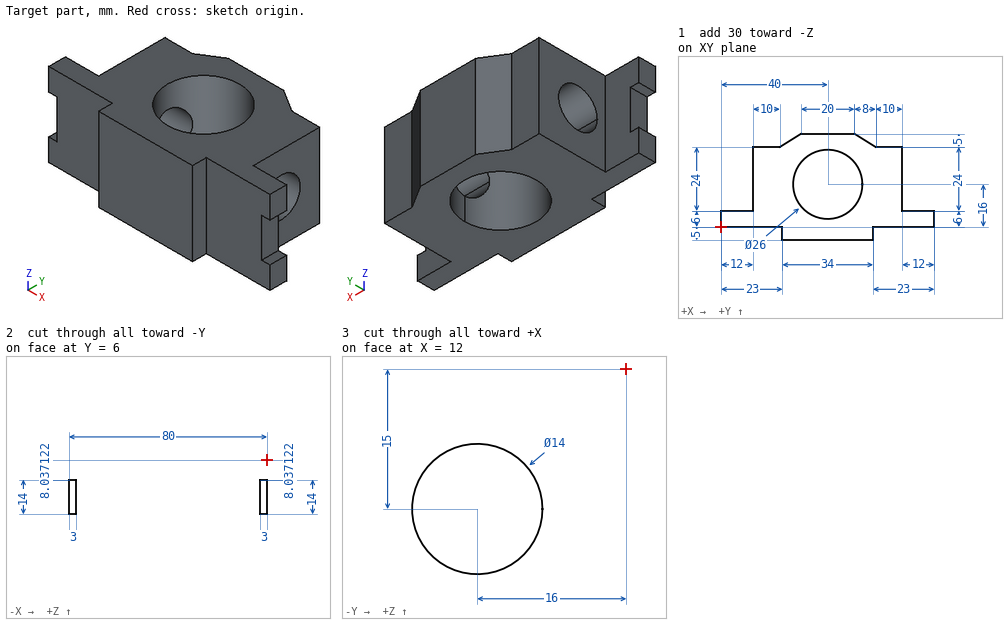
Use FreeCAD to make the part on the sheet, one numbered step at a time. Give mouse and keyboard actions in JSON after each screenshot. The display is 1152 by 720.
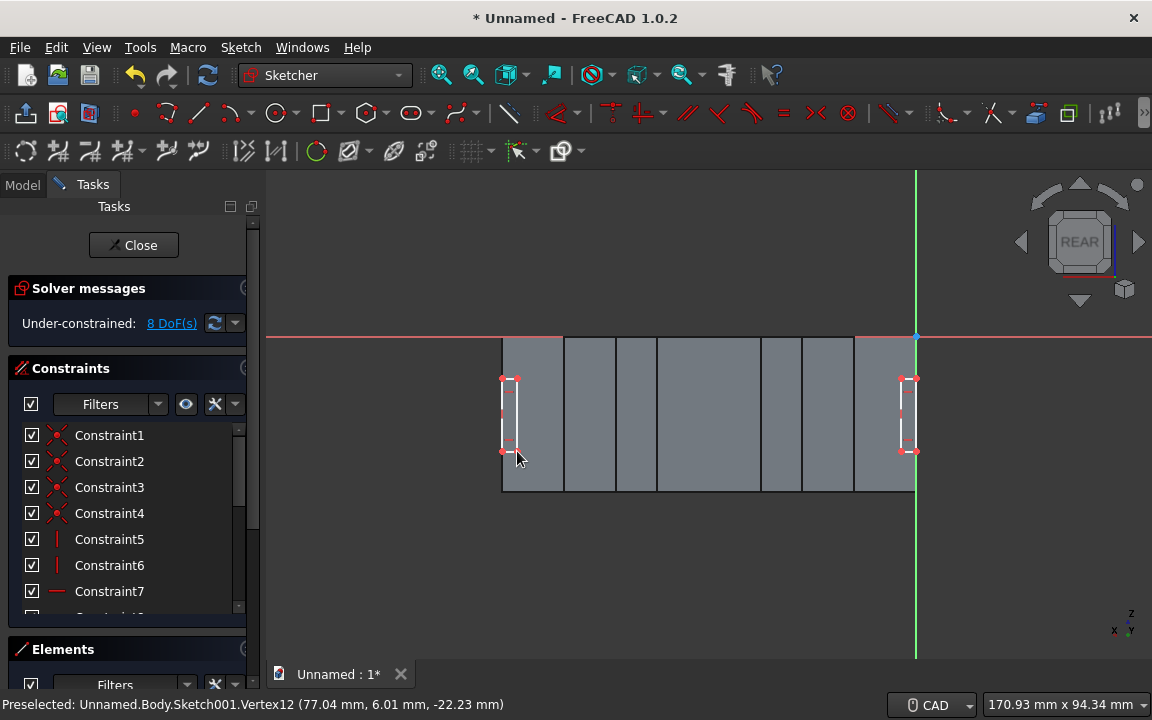
{"action": "left_click", "coordinate": [916, 452]}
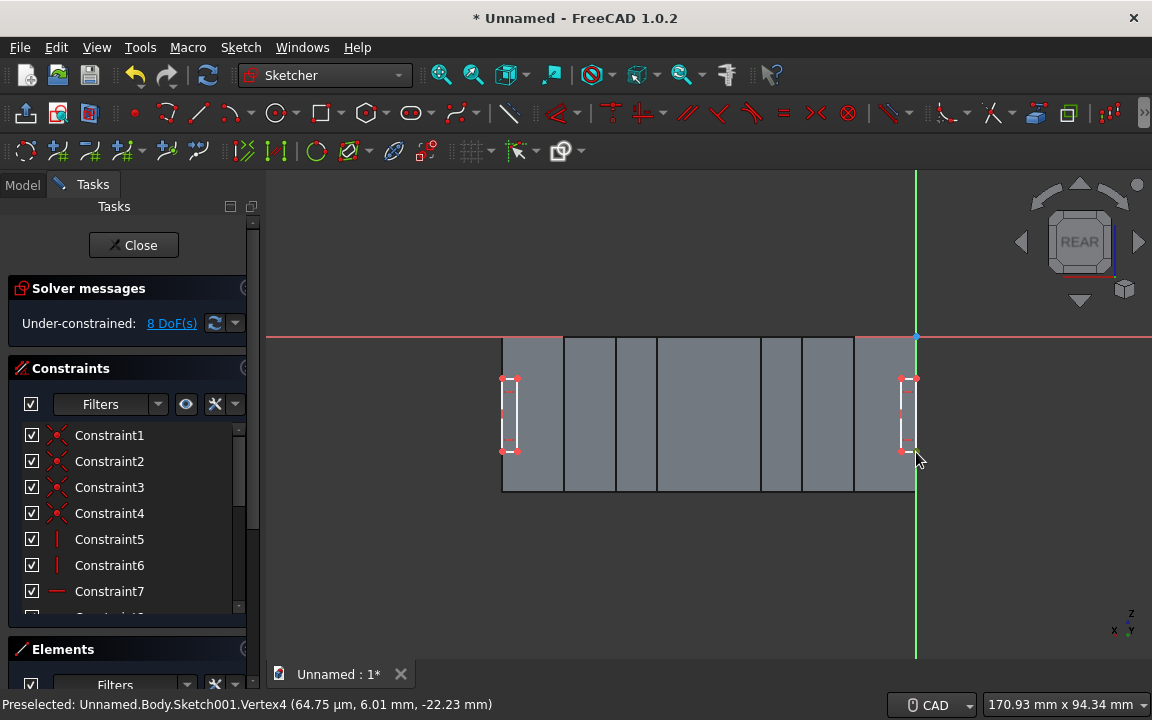
{"action": "left_click", "coordinate": [916, 600]}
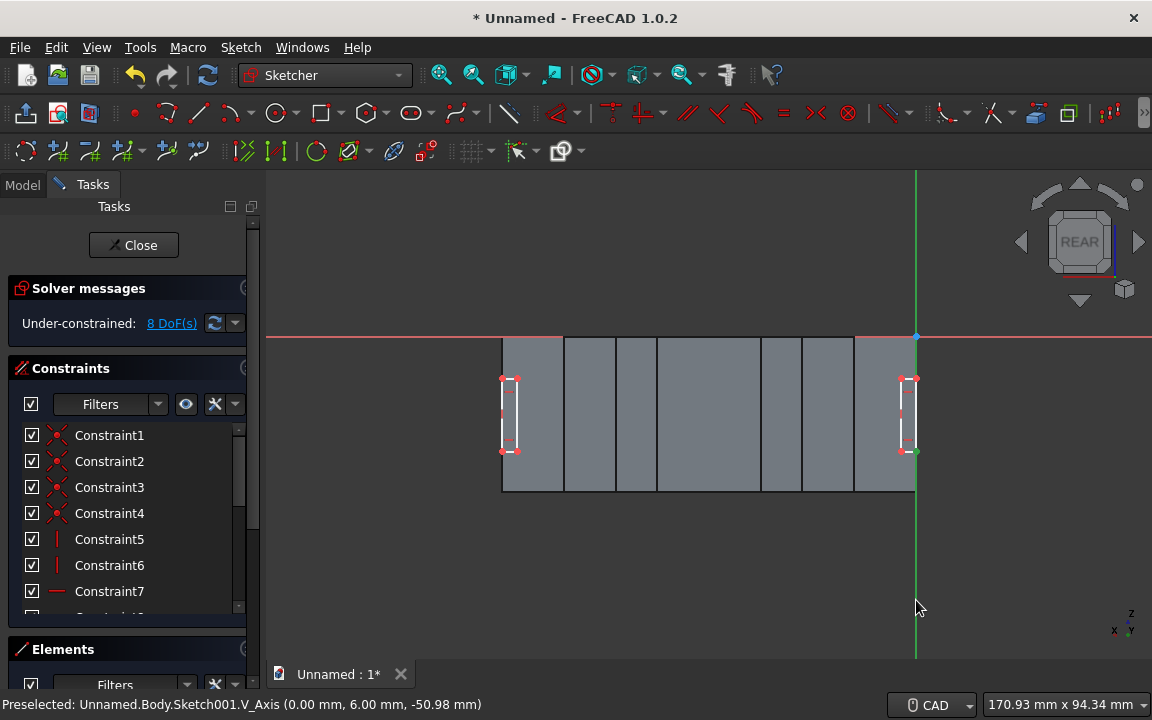
{"action": "key", "text": "c"}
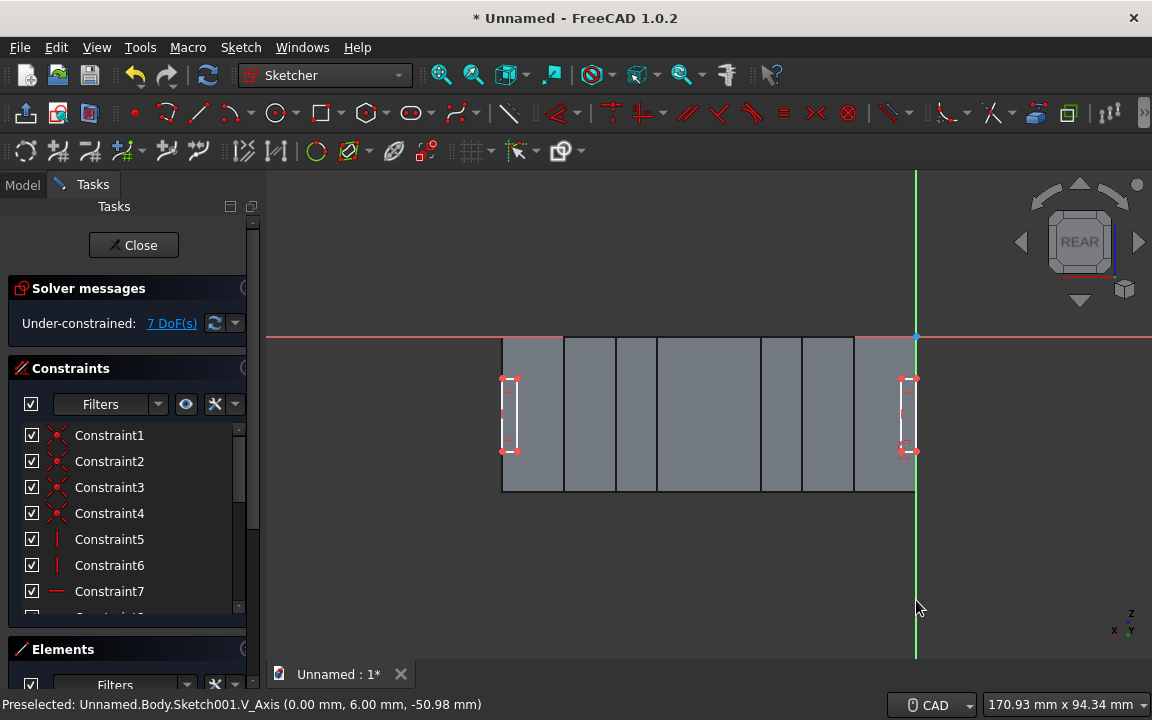
{"action": "left_click", "coordinate": [556, 114]}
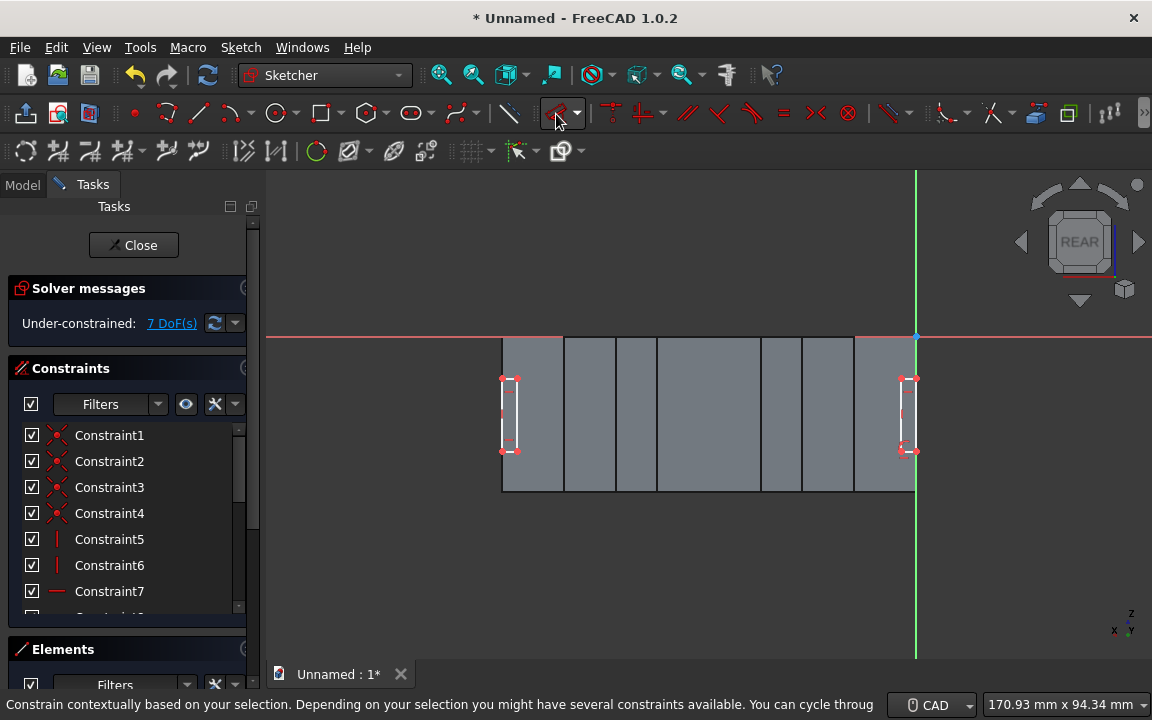
{"action": "scroll", "coordinate": [909, 452], "scroll_direction": "up", "scroll_amount": 5}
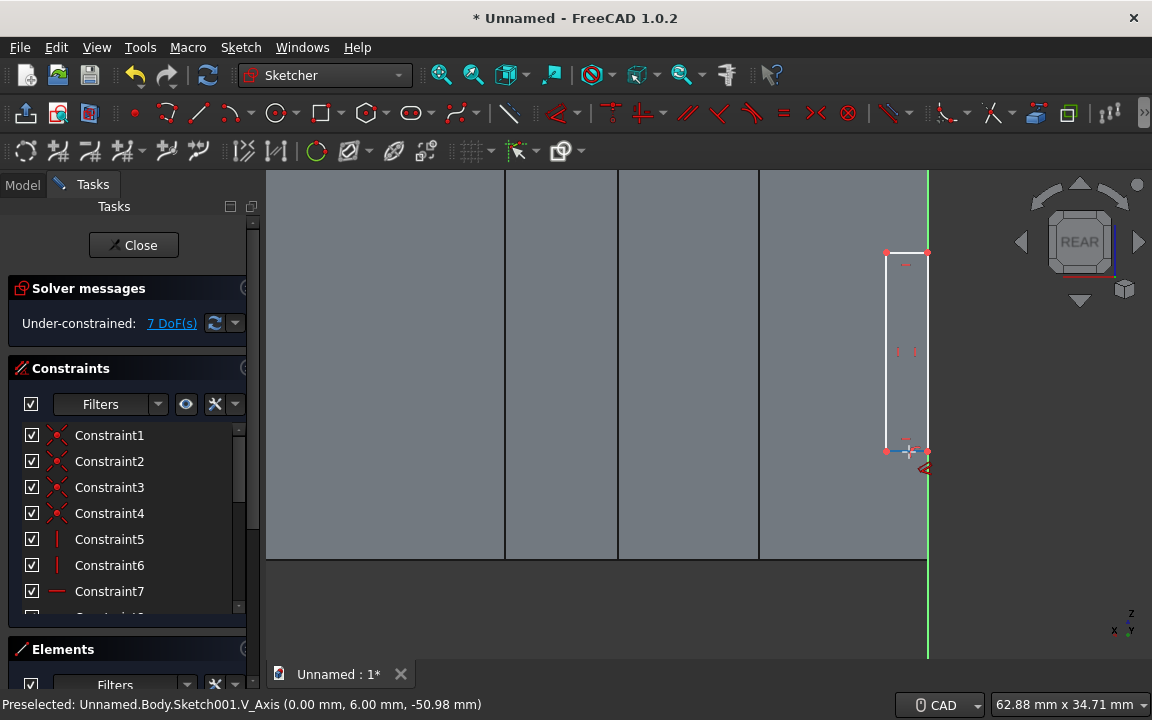
{"action": "left_click", "coordinate": [907, 451]}
{"action": "left_click", "coordinate": [907, 485]}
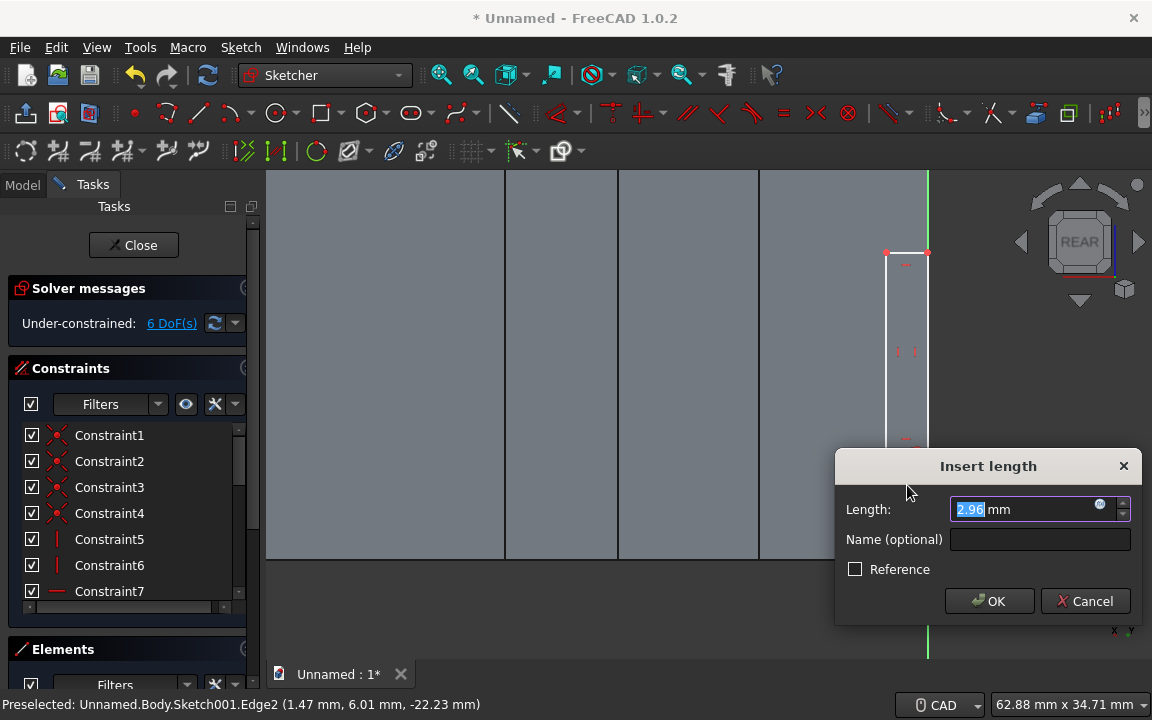
{"action": "type", "text": "3"}
{"action": "key", "text": "Return"}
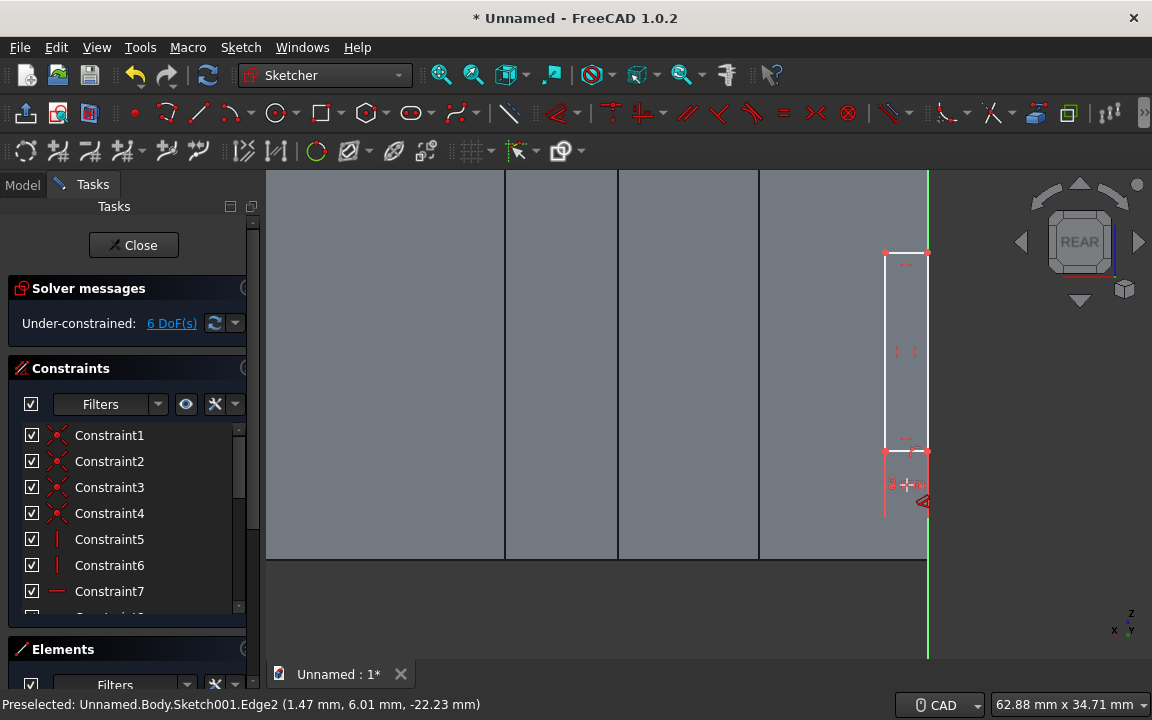
{"action": "scroll", "coordinate": [866, 514], "scroll_direction": "down", "scroll_amount": 4}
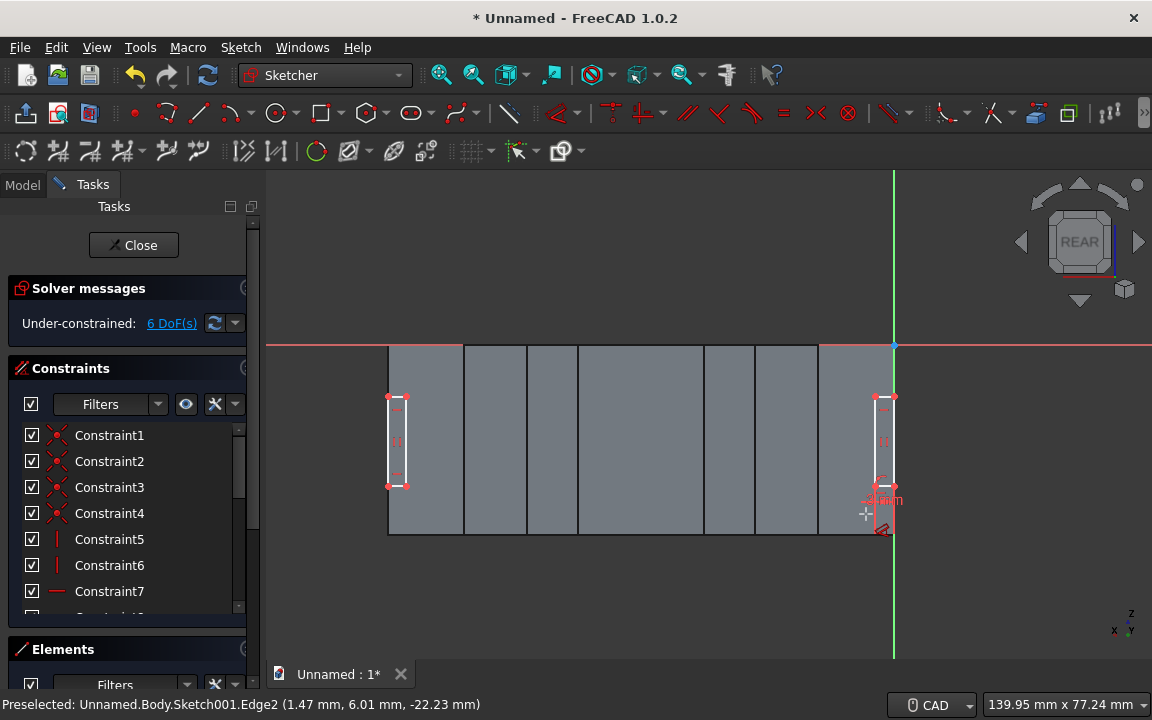
{"action": "scroll", "coordinate": [394, 486], "scroll_direction": "up", "scroll_amount": 5}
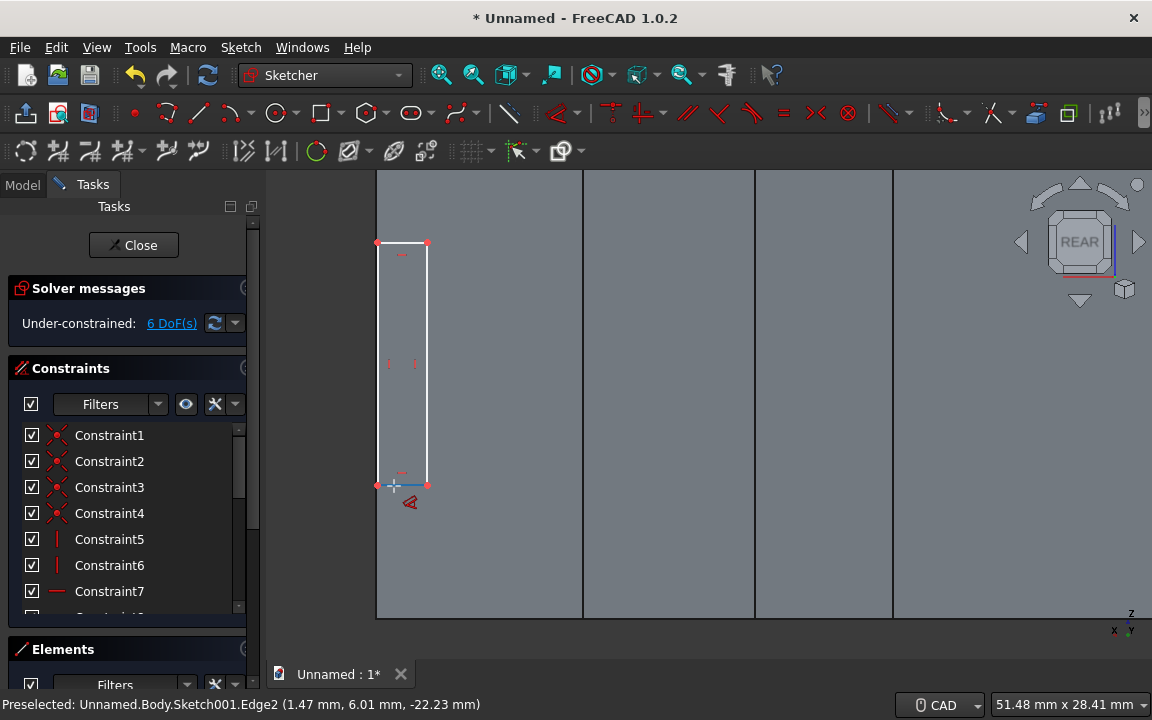
{"action": "left_click", "coordinate": [392, 485]}
{"action": "left_click", "coordinate": [402, 519]}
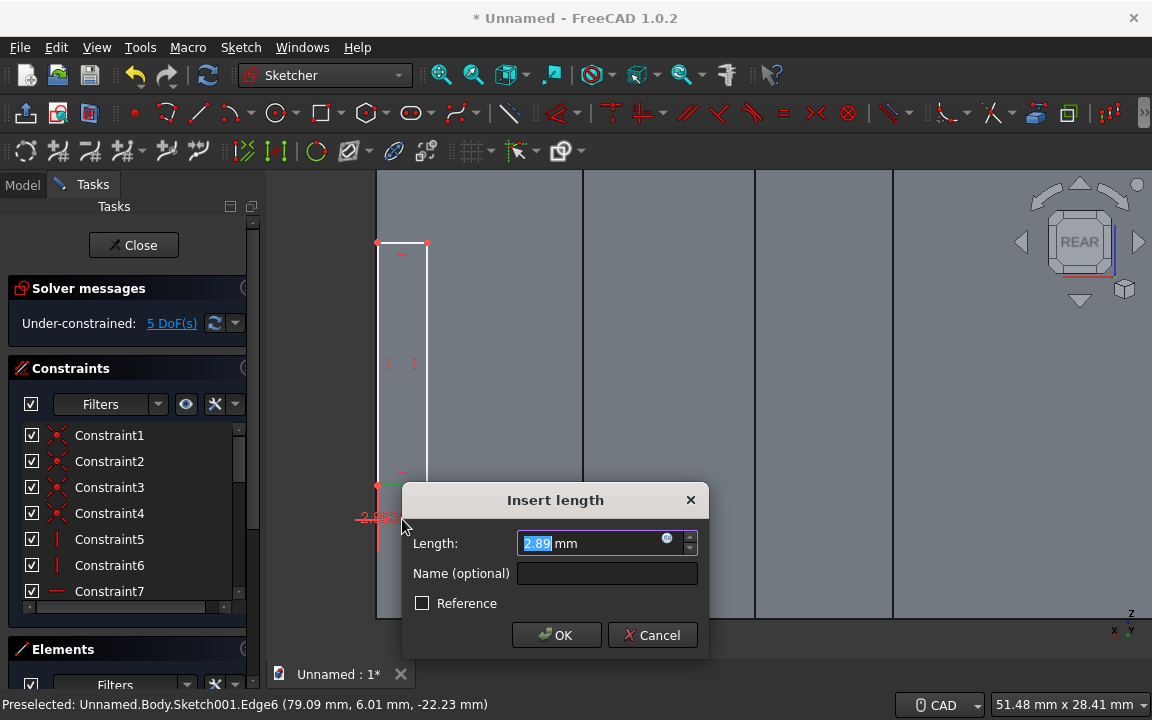
{"action": "type", "text": "3"}
{"action": "key", "text": "Return"}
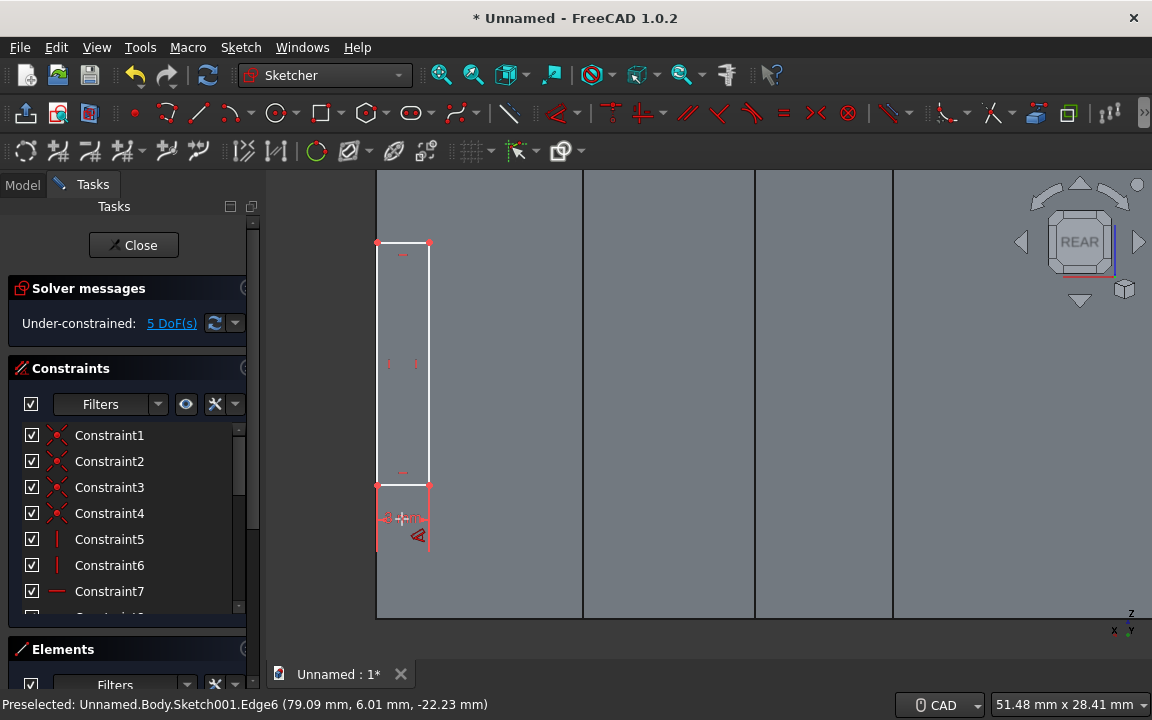
{"action": "scroll", "coordinate": [394, 486], "scroll_direction": "down", "scroll_amount": 5}